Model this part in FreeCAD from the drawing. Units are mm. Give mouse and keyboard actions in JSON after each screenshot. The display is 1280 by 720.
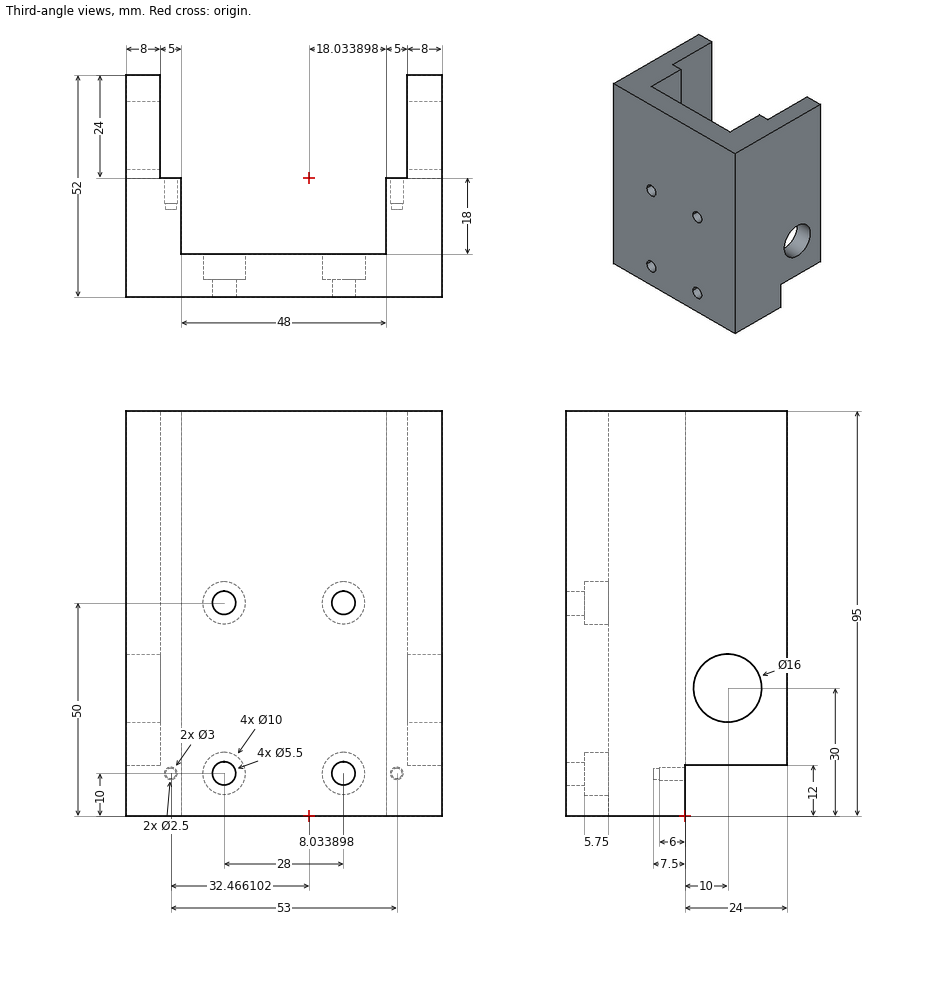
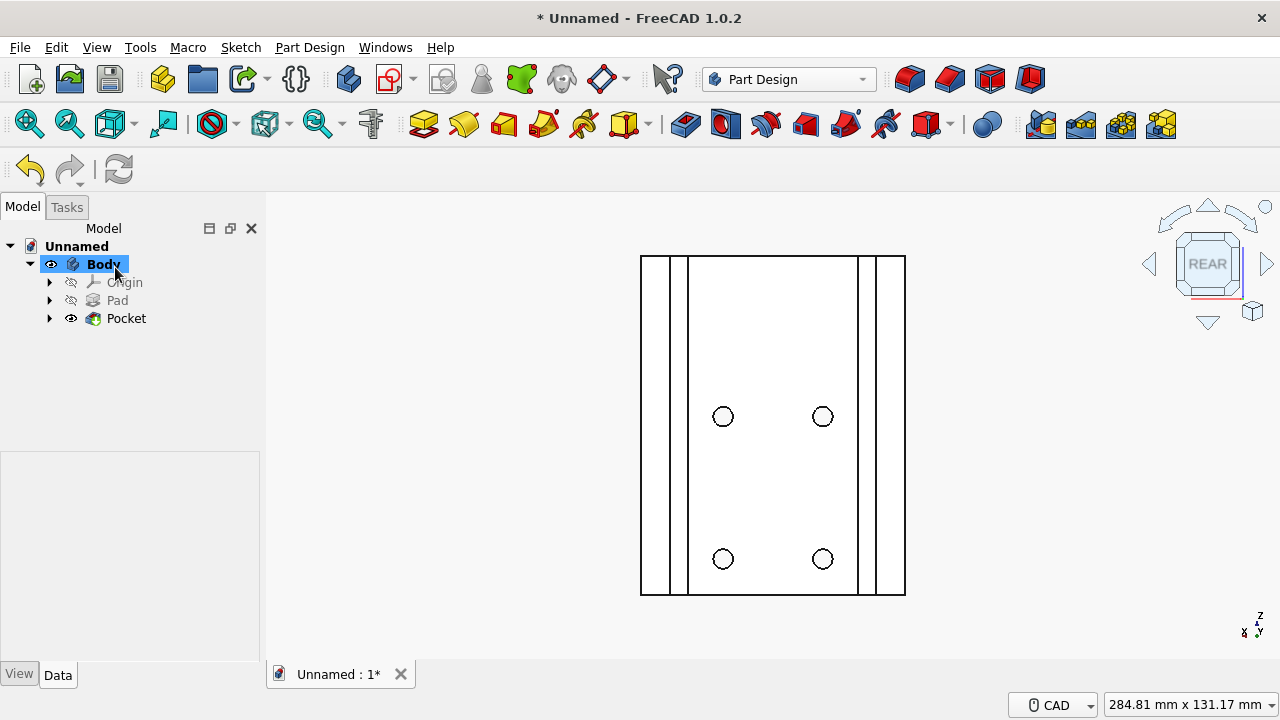
{"action": "left_click", "coordinate": [773, 328]}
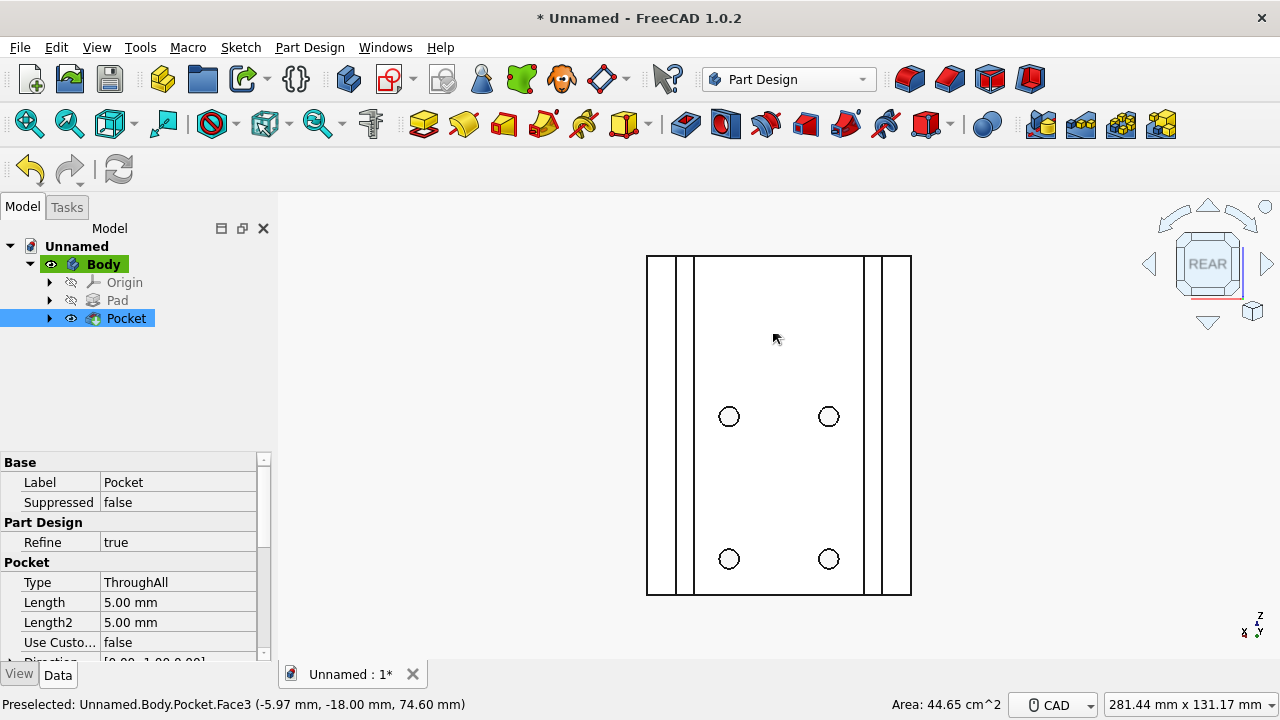
{"action": "left_click", "coordinate": [390, 80]}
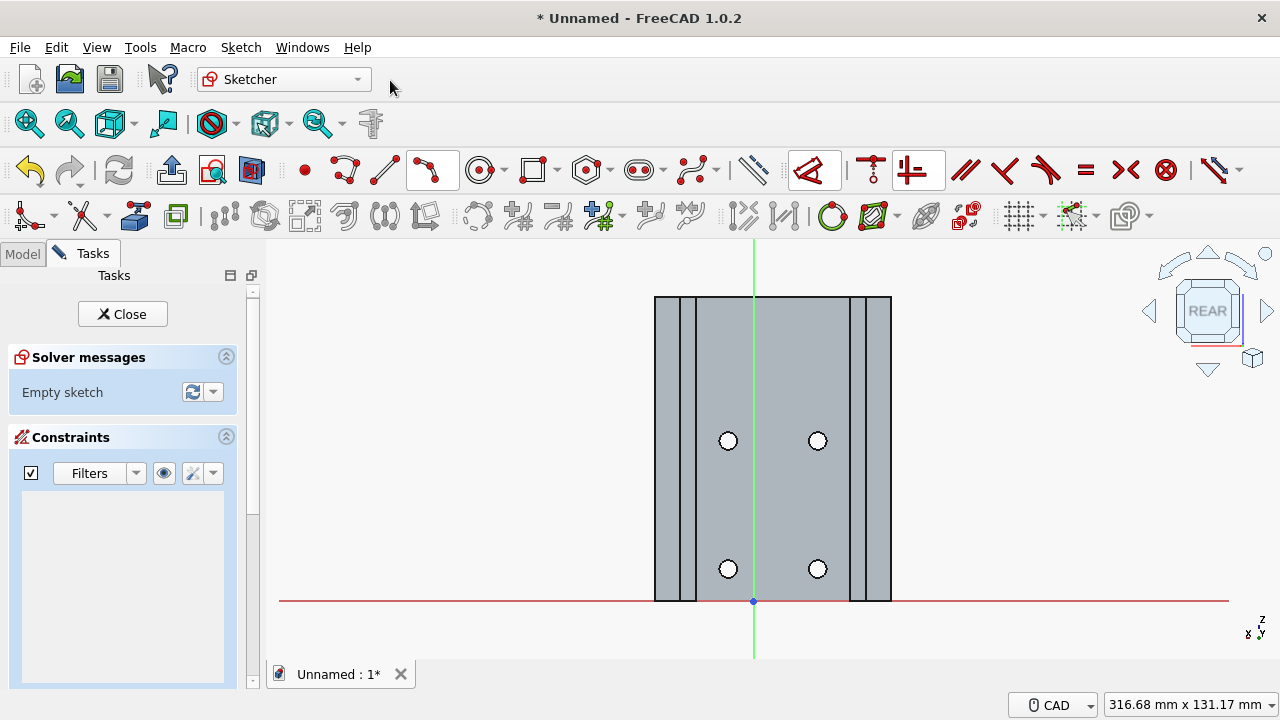
{"action": "key", "text": "q s"}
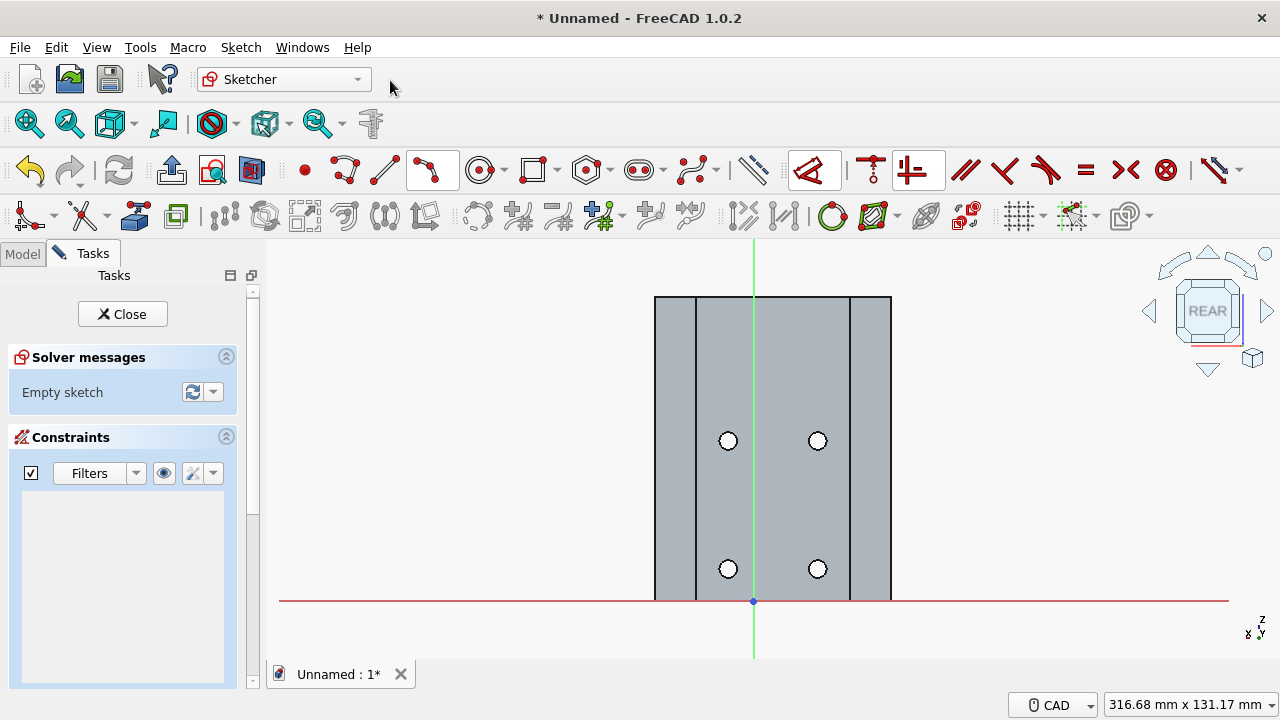
{"action": "scroll", "coordinate": [912, 631], "scroll_direction": "up", "scroll_amount": 2}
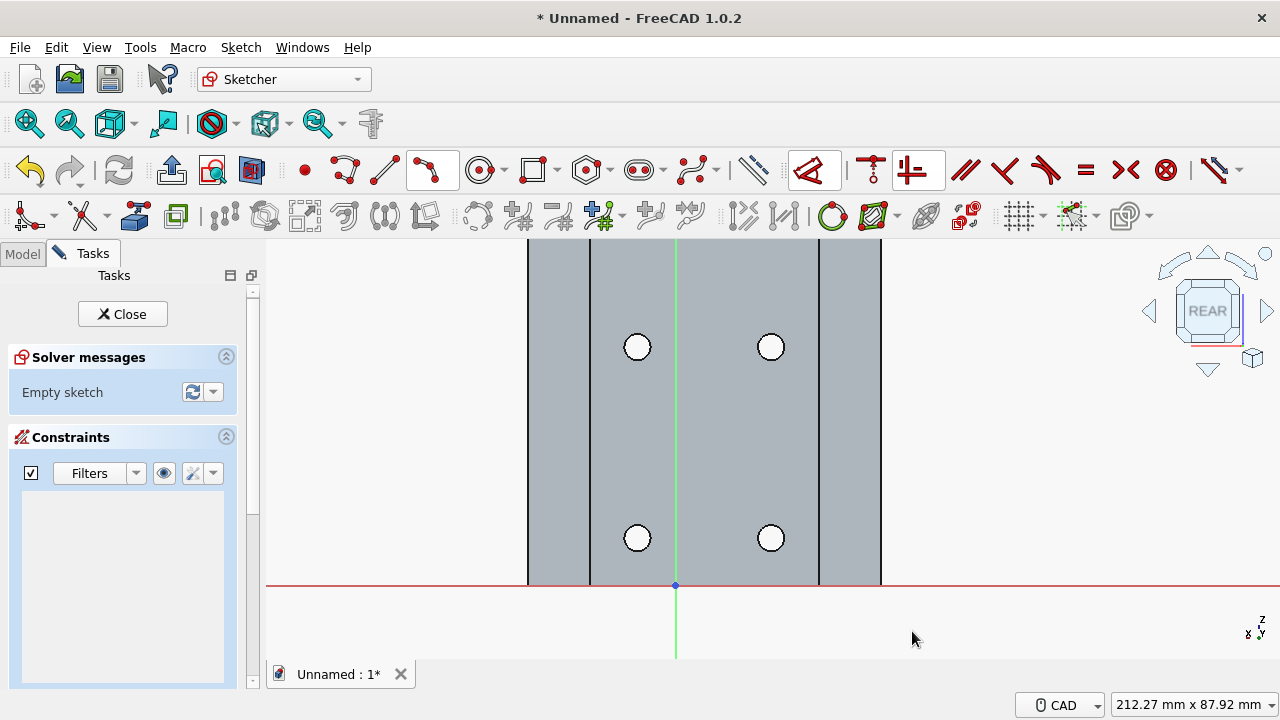
{"action": "key", "text": "g c"}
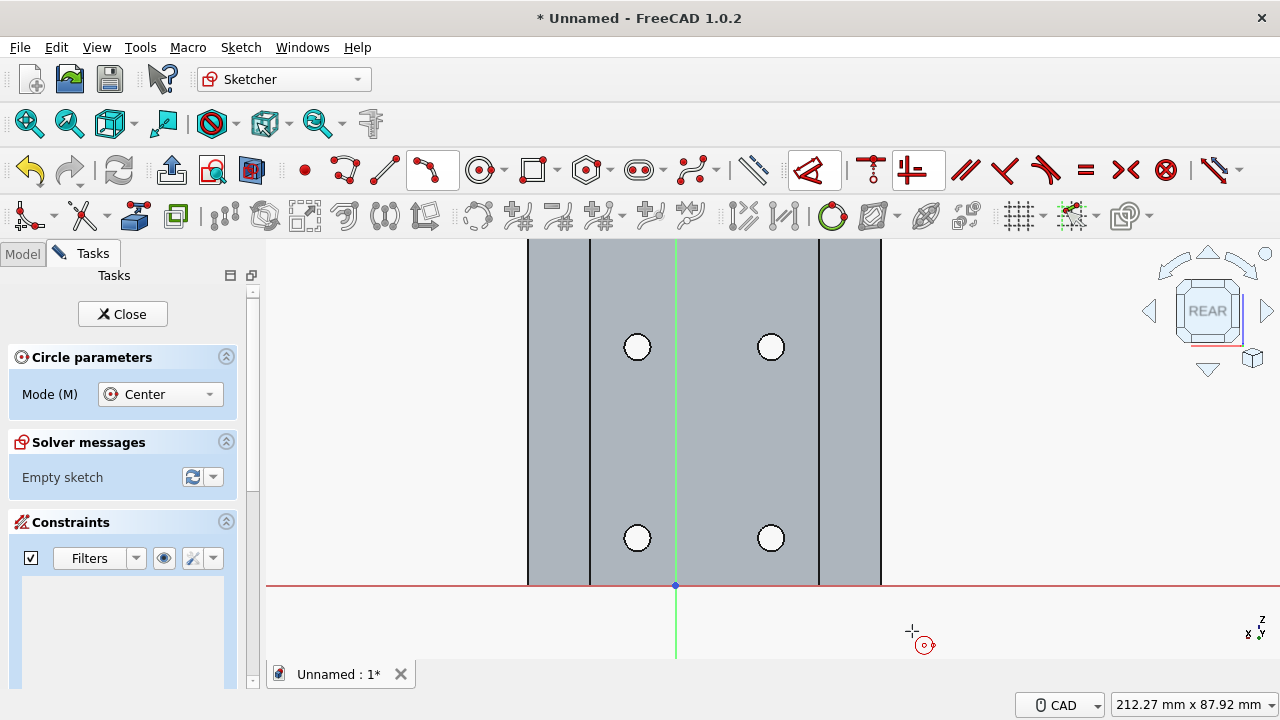
{"action": "left_click", "coordinate": [771, 538]}
{"action": "left_click", "coordinate": [788, 521]}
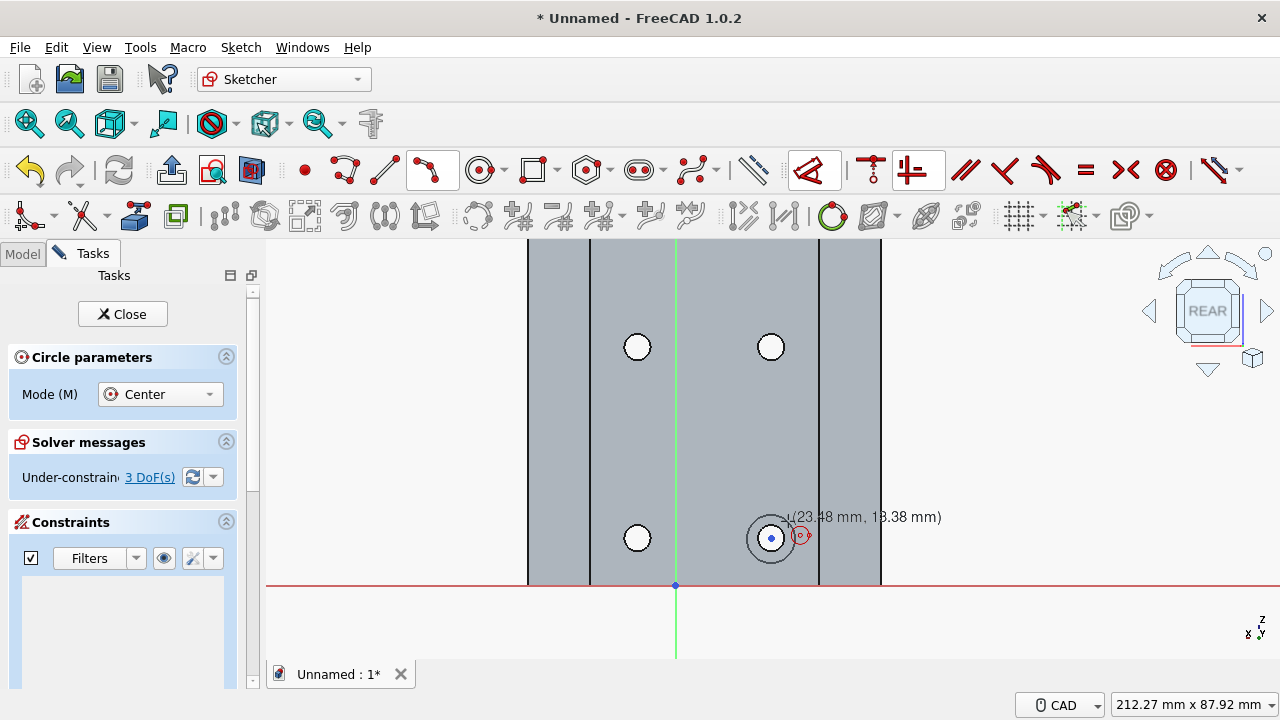
{"action": "left_click", "coordinate": [771, 347]}
{"action": "left_click", "coordinate": [788, 330]}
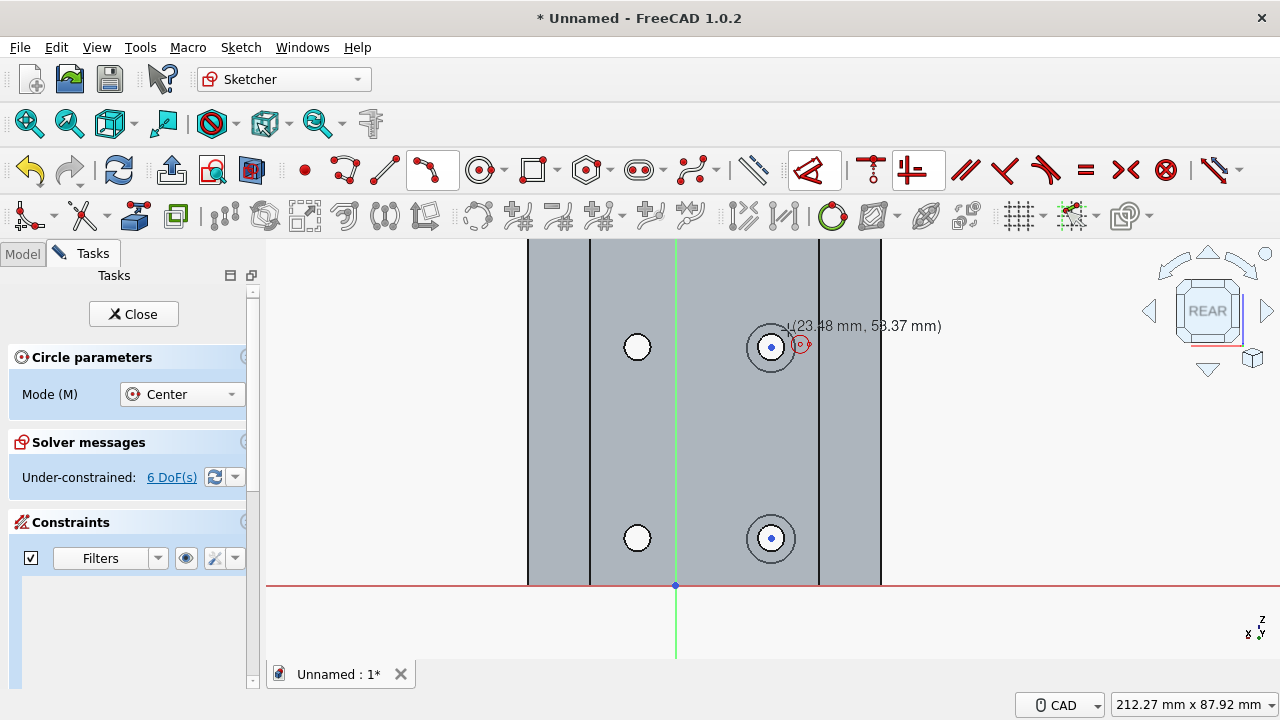
{"action": "left_click", "coordinate": [637, 538]}
{"action": "left_click", "coordinate": [654, 521]}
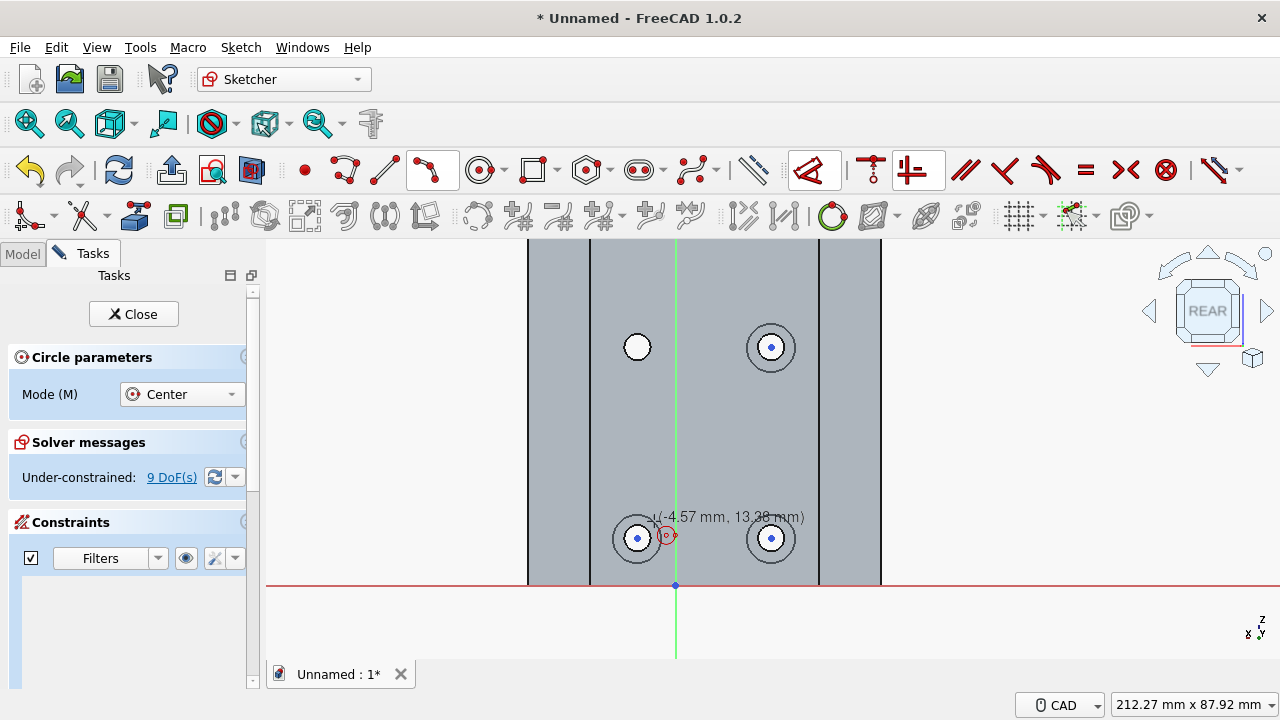
{"action": "left_click", "coordinate": [637, 347]}
{"action": "left_click", "coordinate": [654, 330]}
{"action": "key", "text": "Escape"}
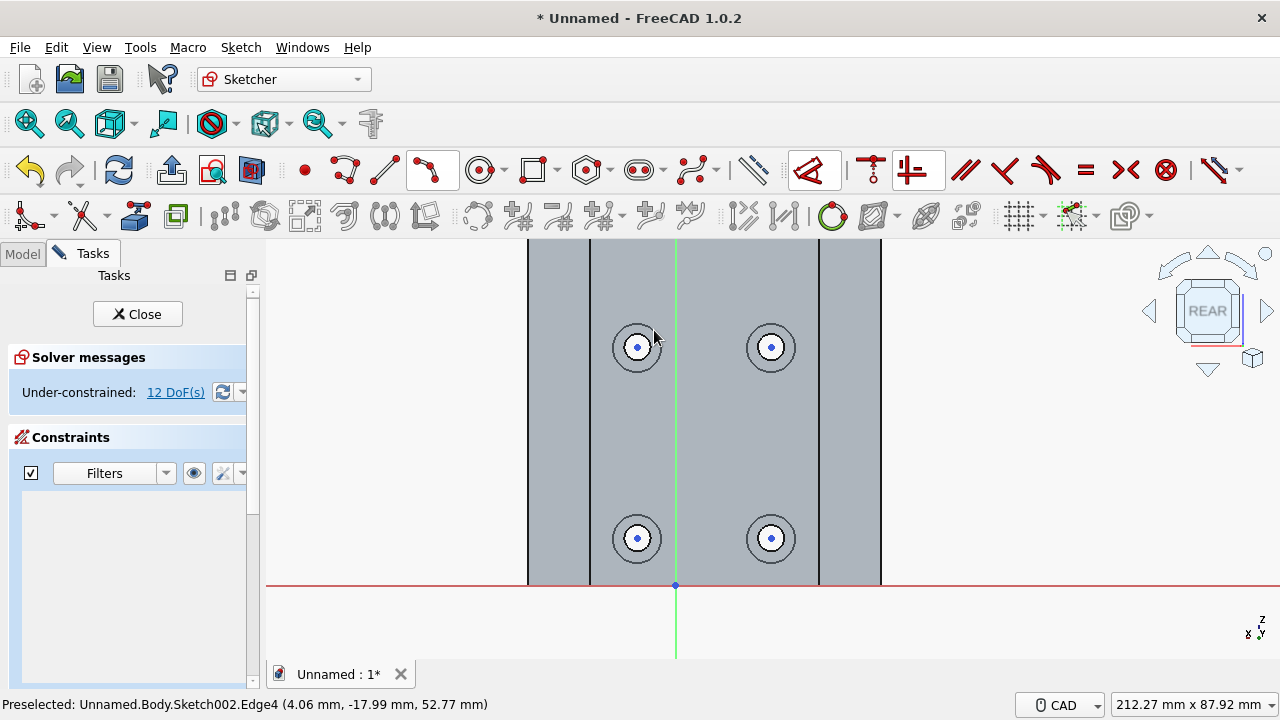
{"action": "left_click", "coordinate": [788, 522]}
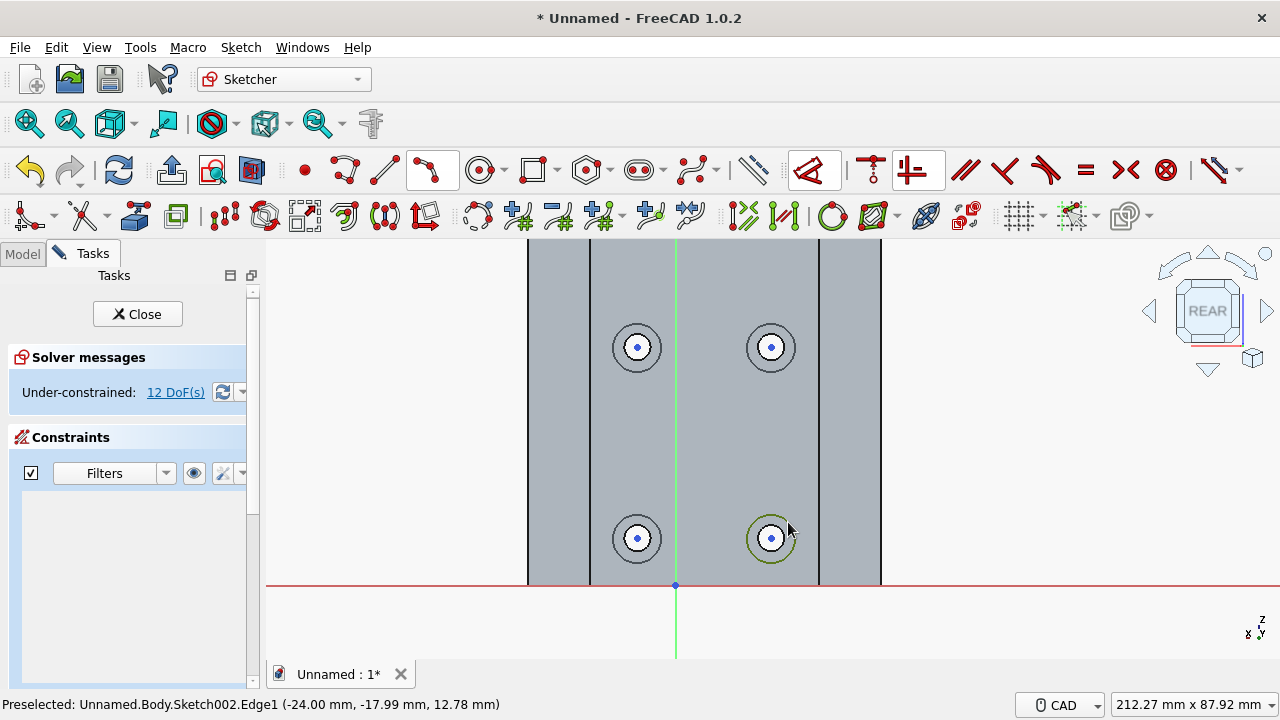
{"action": "left_click", "coordinate": [788, 331]}